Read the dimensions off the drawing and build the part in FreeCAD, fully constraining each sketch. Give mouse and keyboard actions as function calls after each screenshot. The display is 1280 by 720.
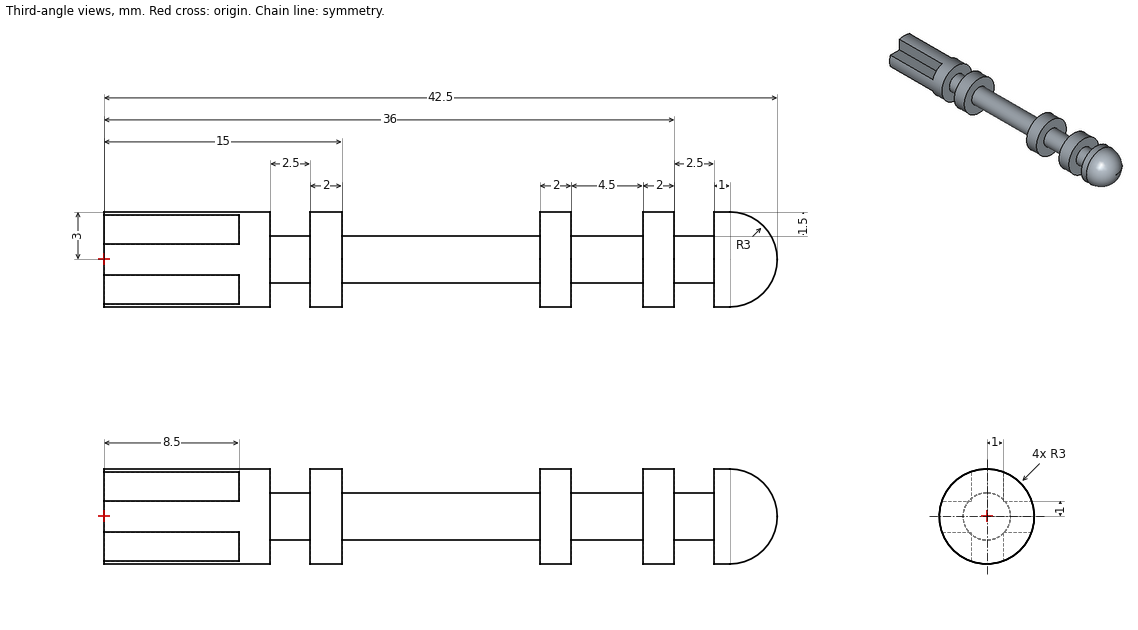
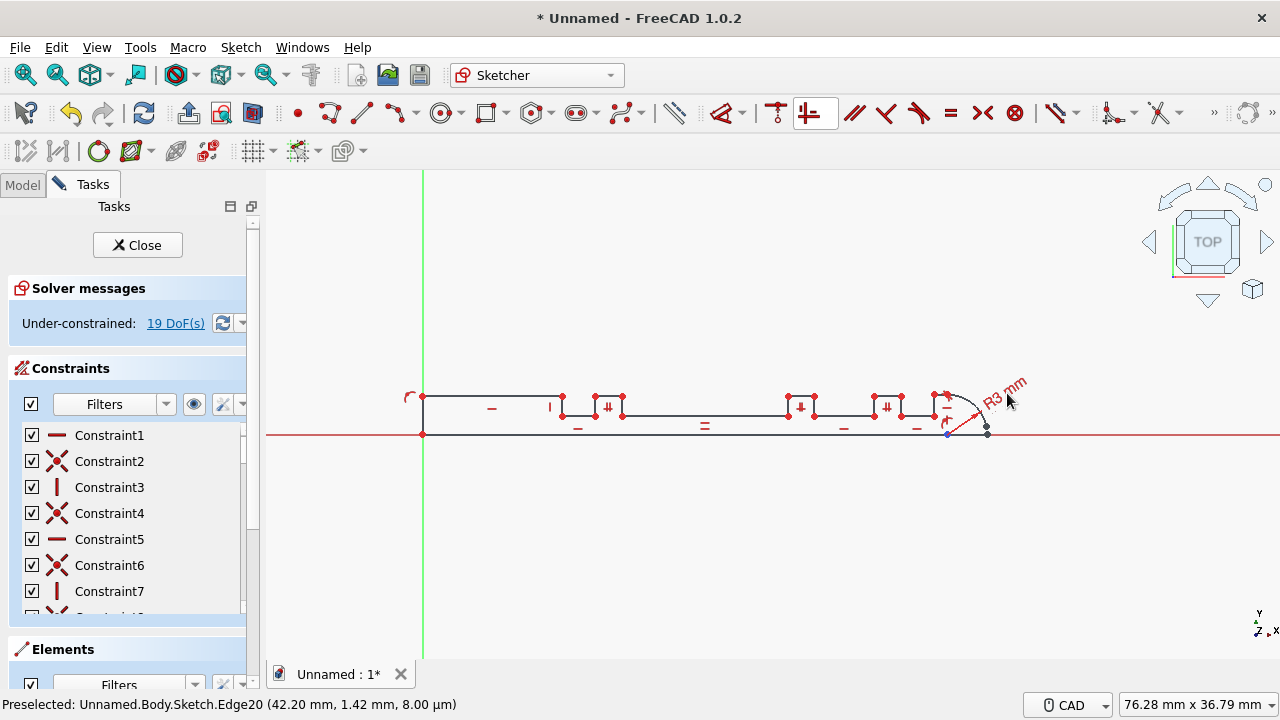
click(986, 426)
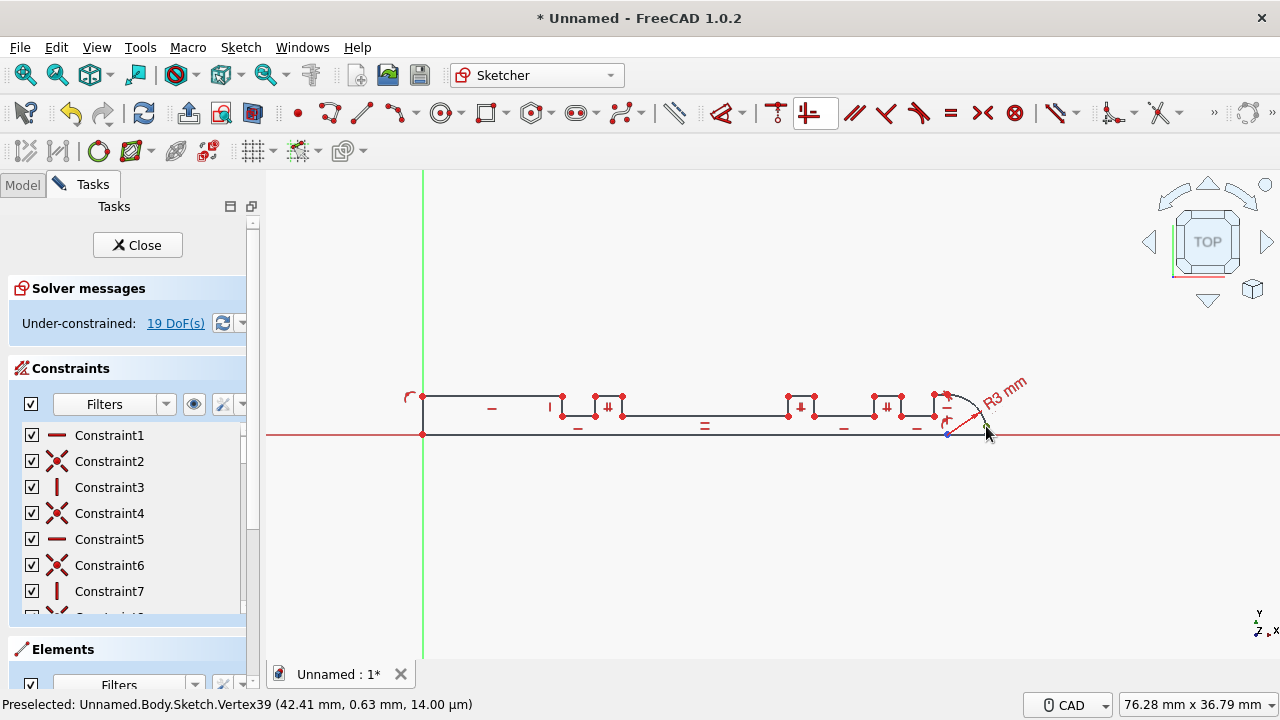
click(353, 435)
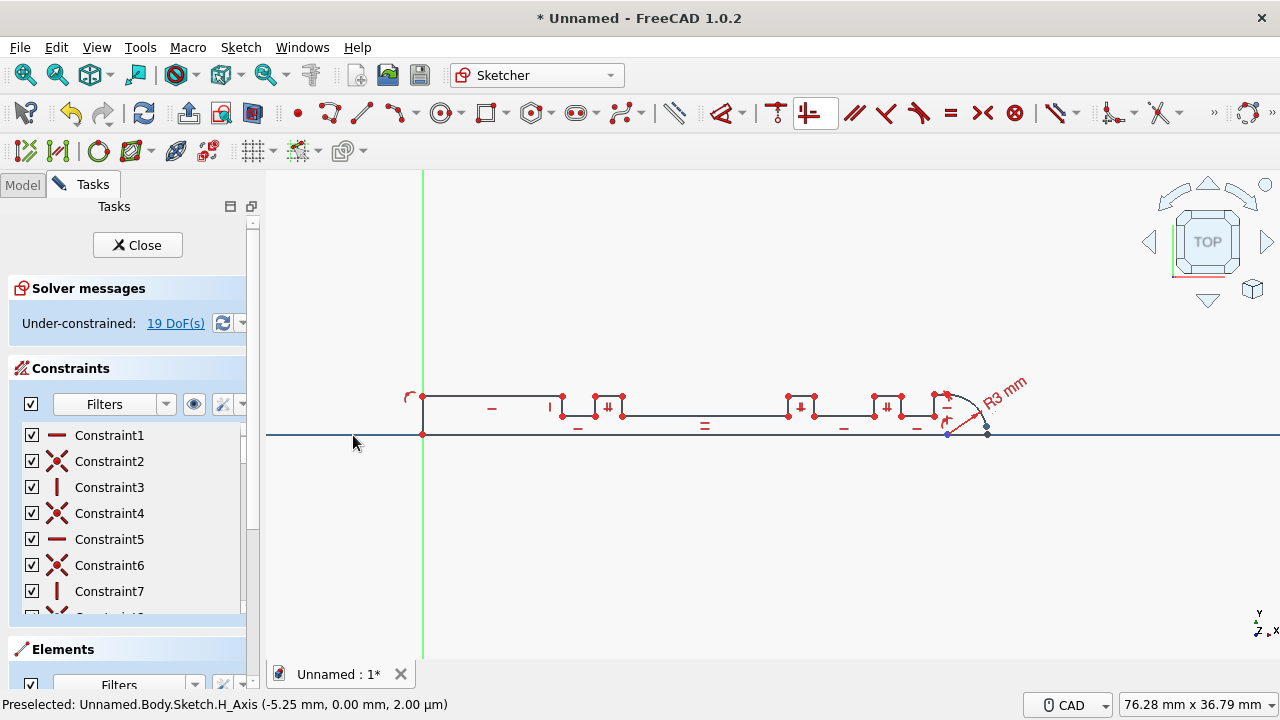
click(776, 114)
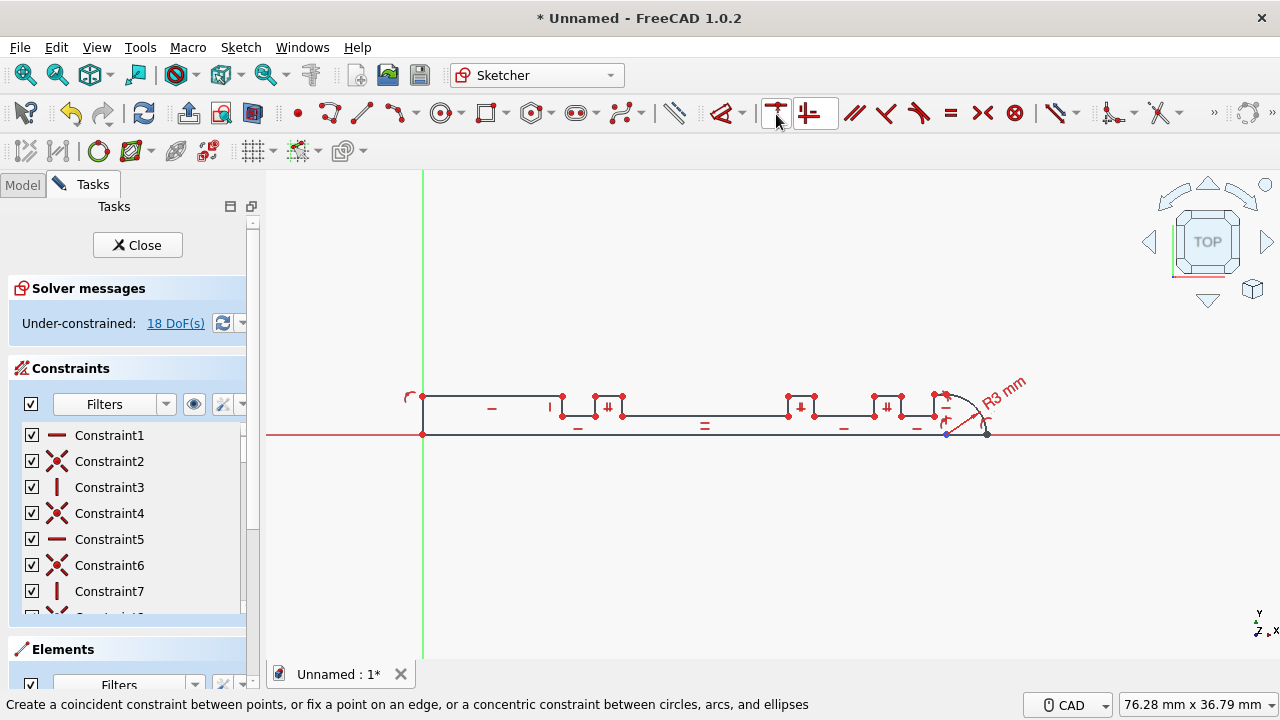
click(722, 114)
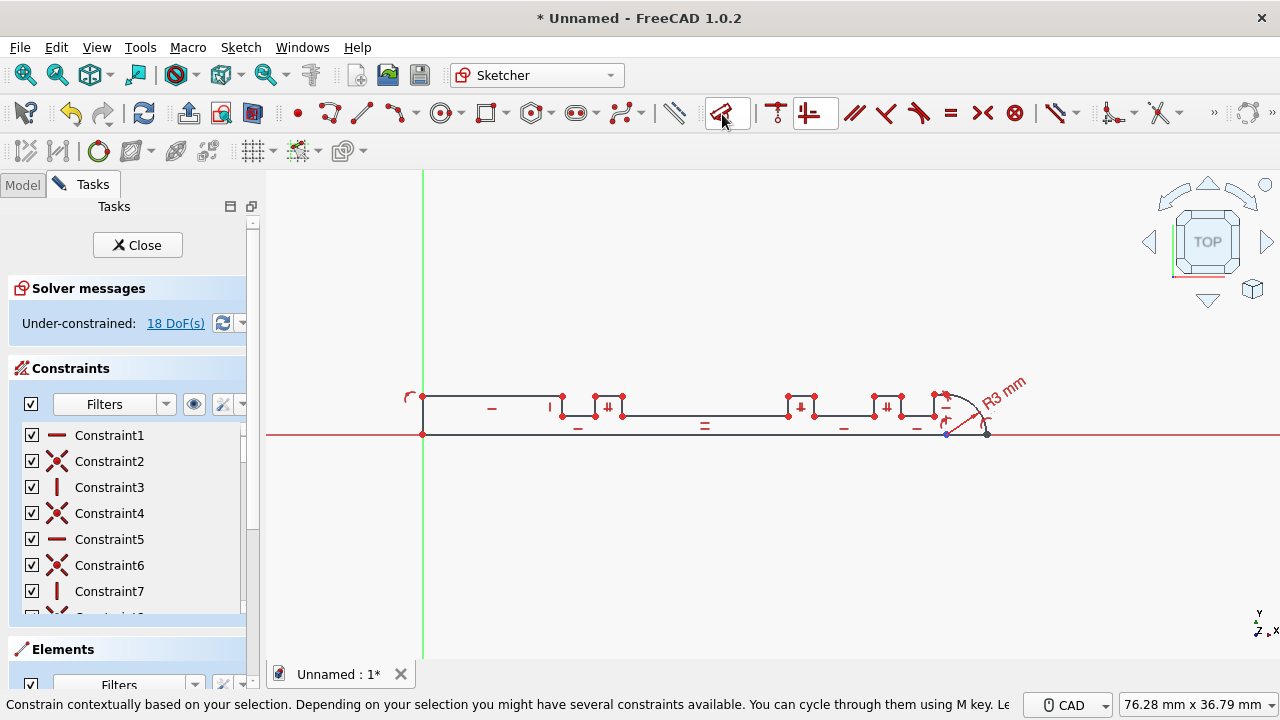
scroll(941, 395, up, 6)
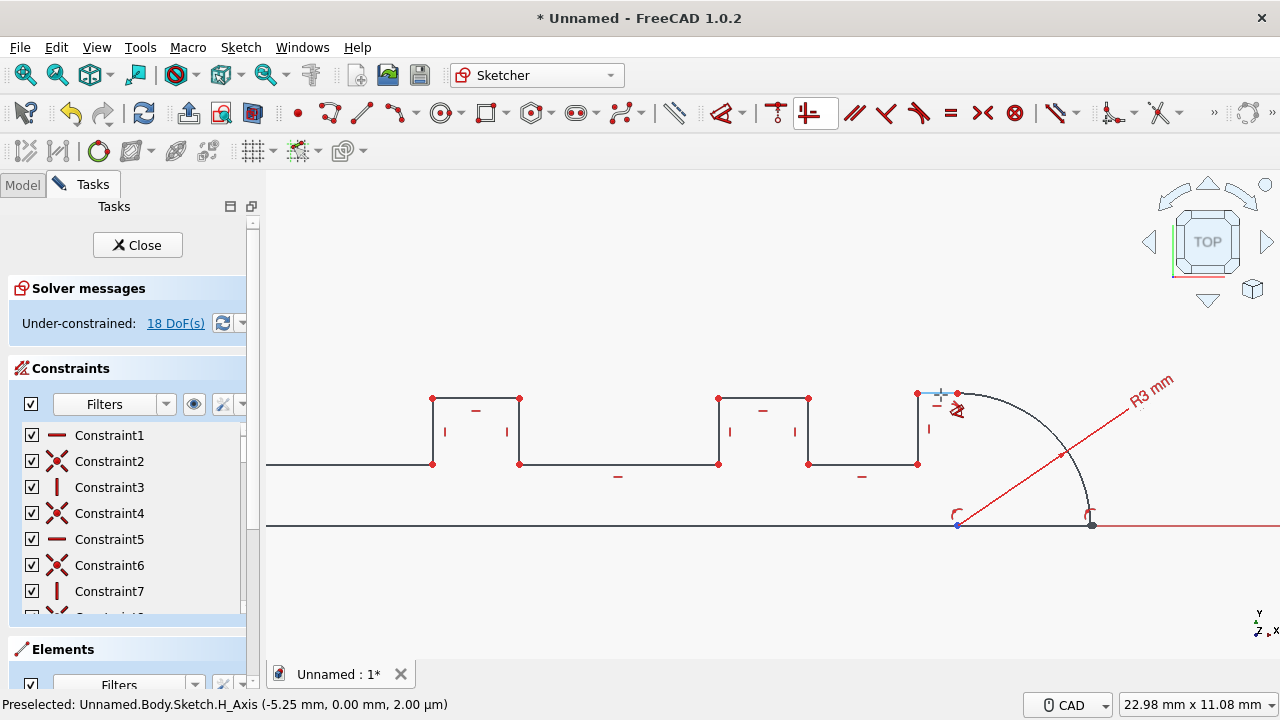
click(938, 393)
click(938, 359)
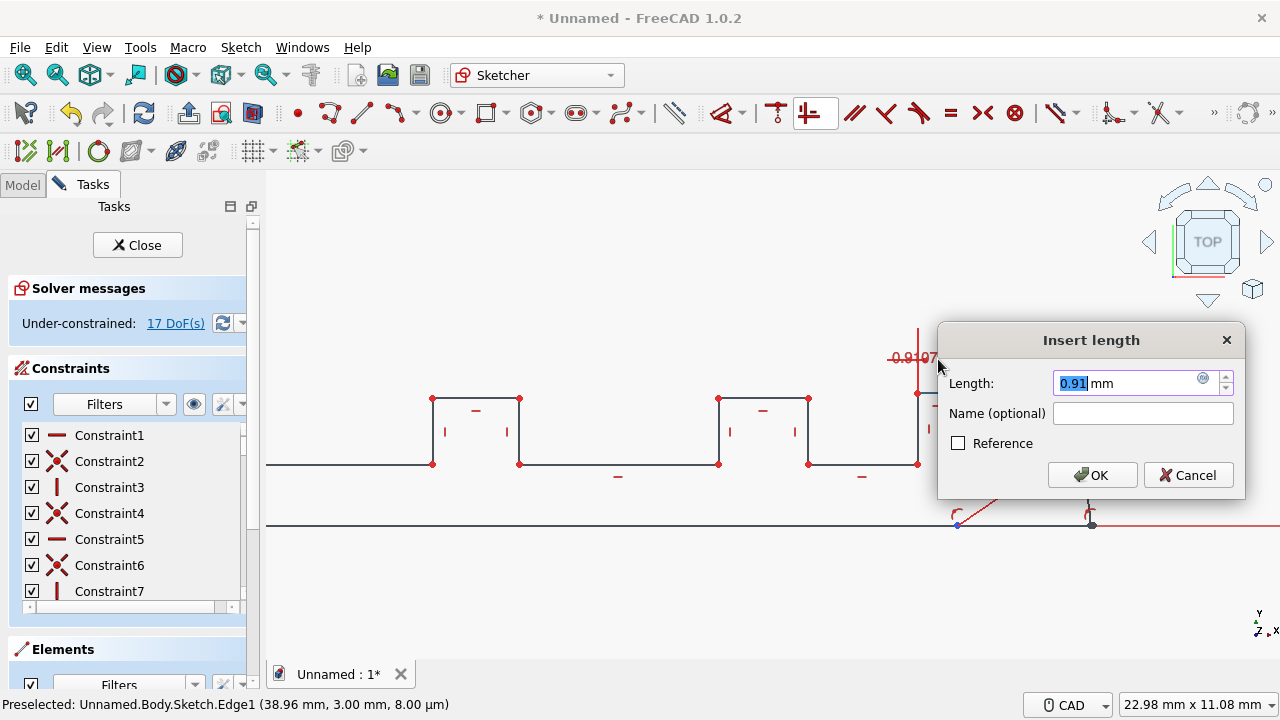
text(1)
key(Return)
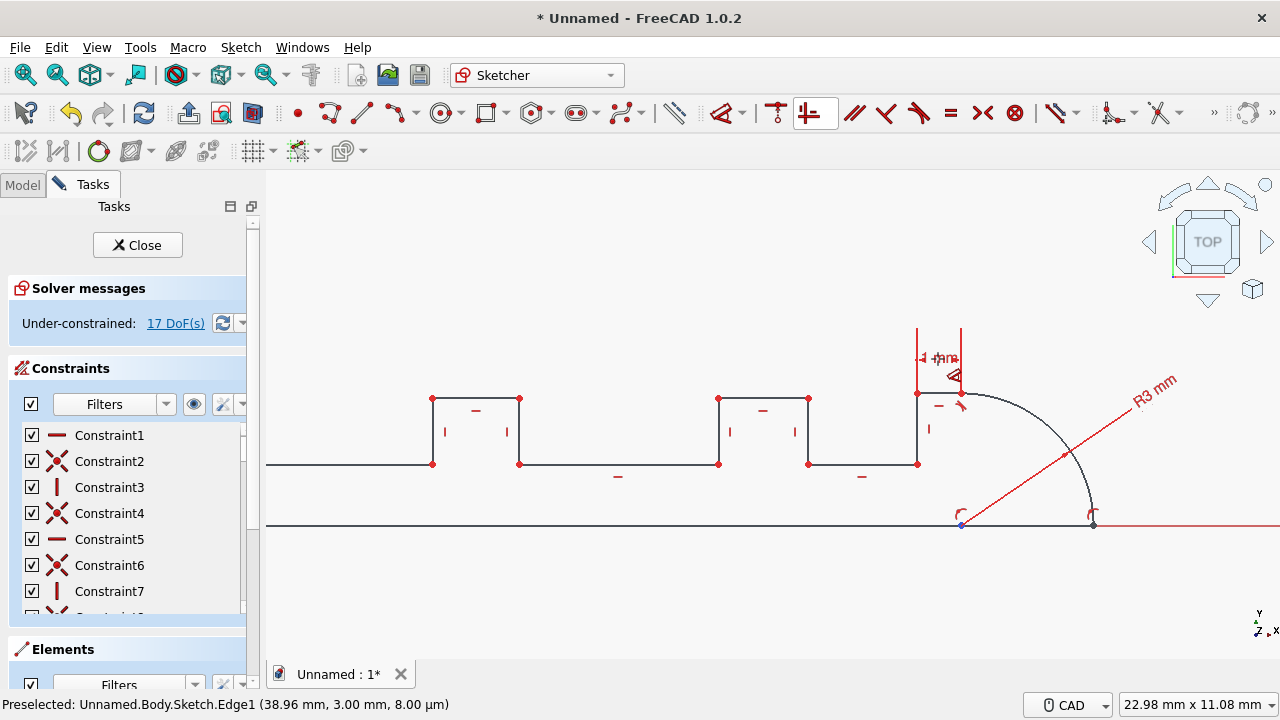
click(781, 398)
click(763, 364)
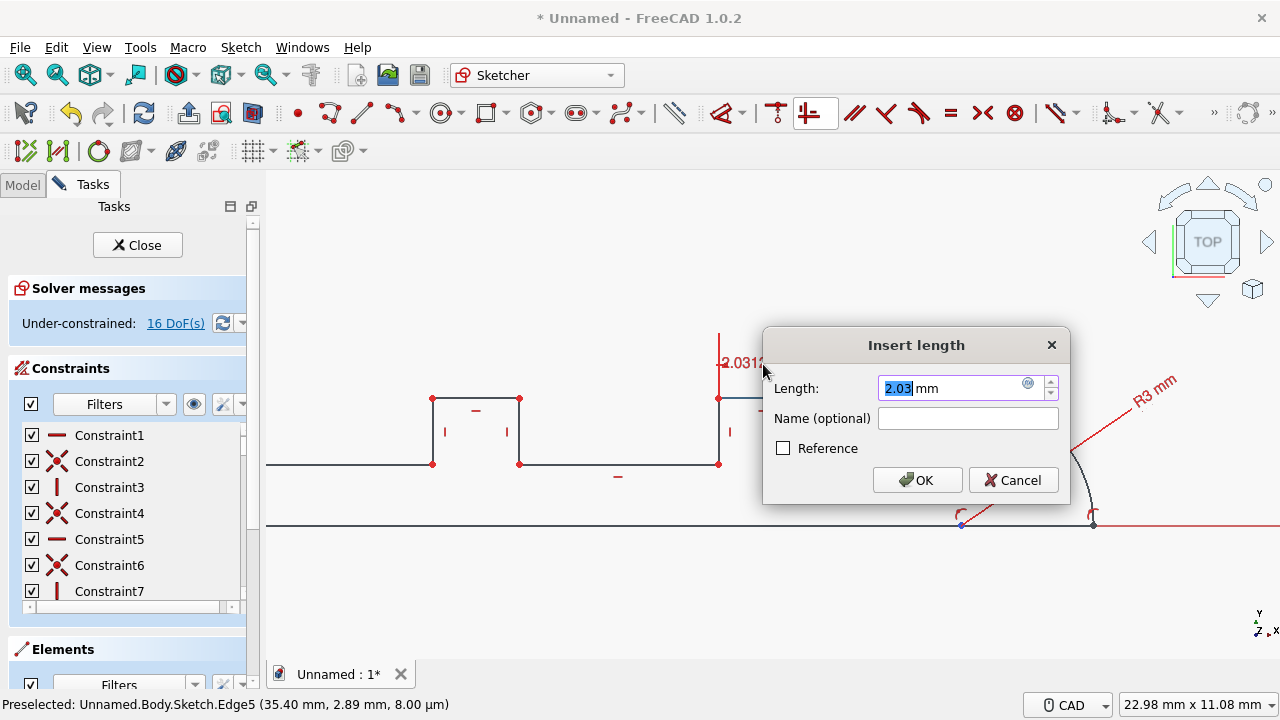
text(2)
key(Return)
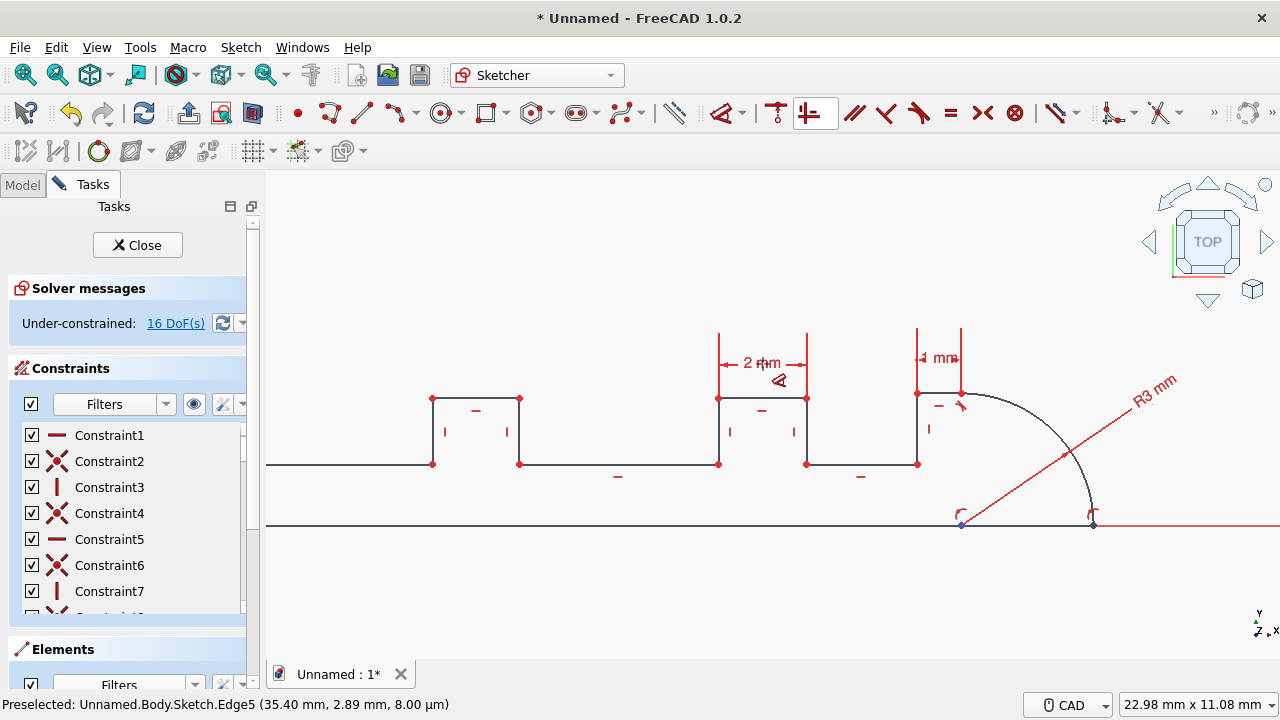
click(493, 398)
click(476, 364)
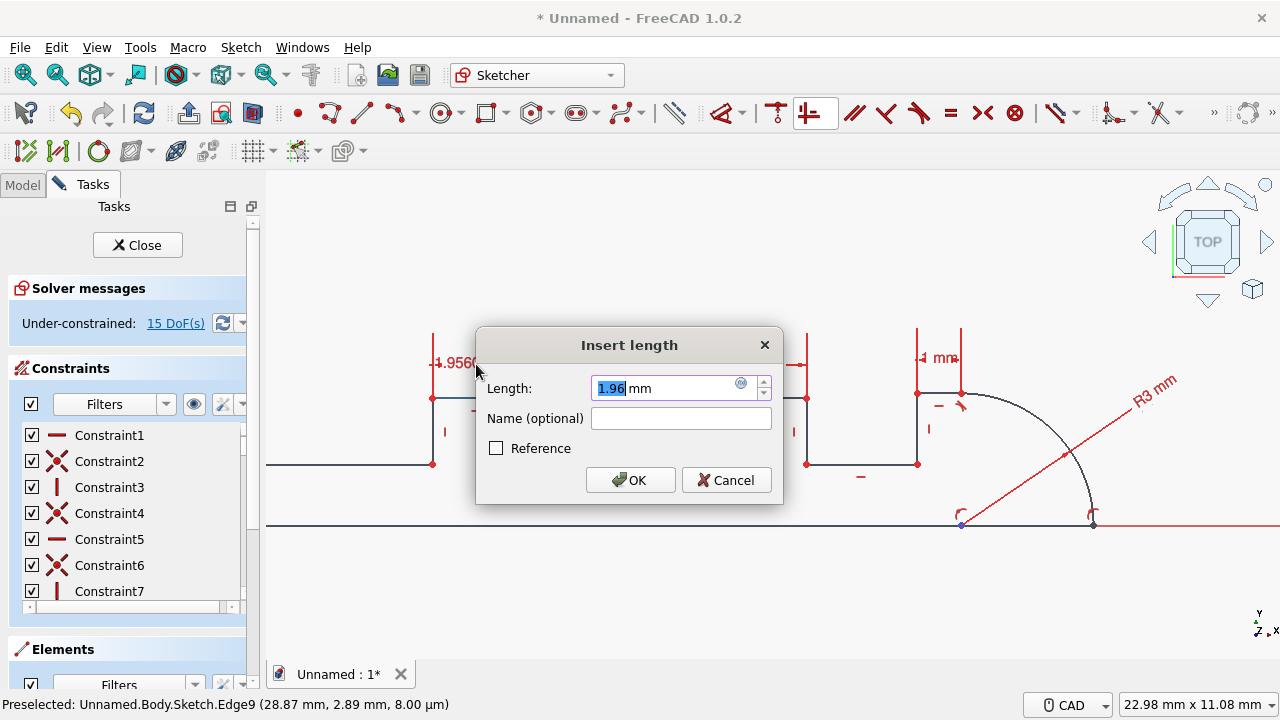
text(2)
key(Return)